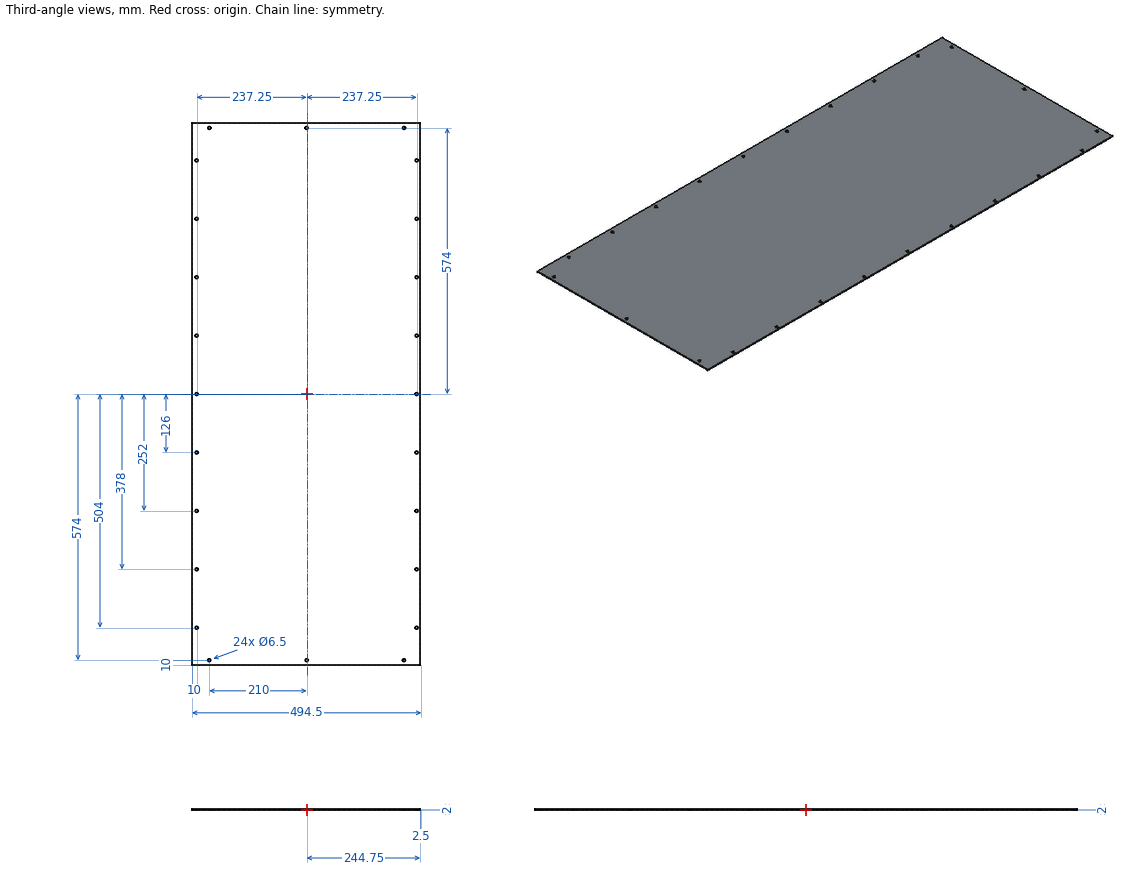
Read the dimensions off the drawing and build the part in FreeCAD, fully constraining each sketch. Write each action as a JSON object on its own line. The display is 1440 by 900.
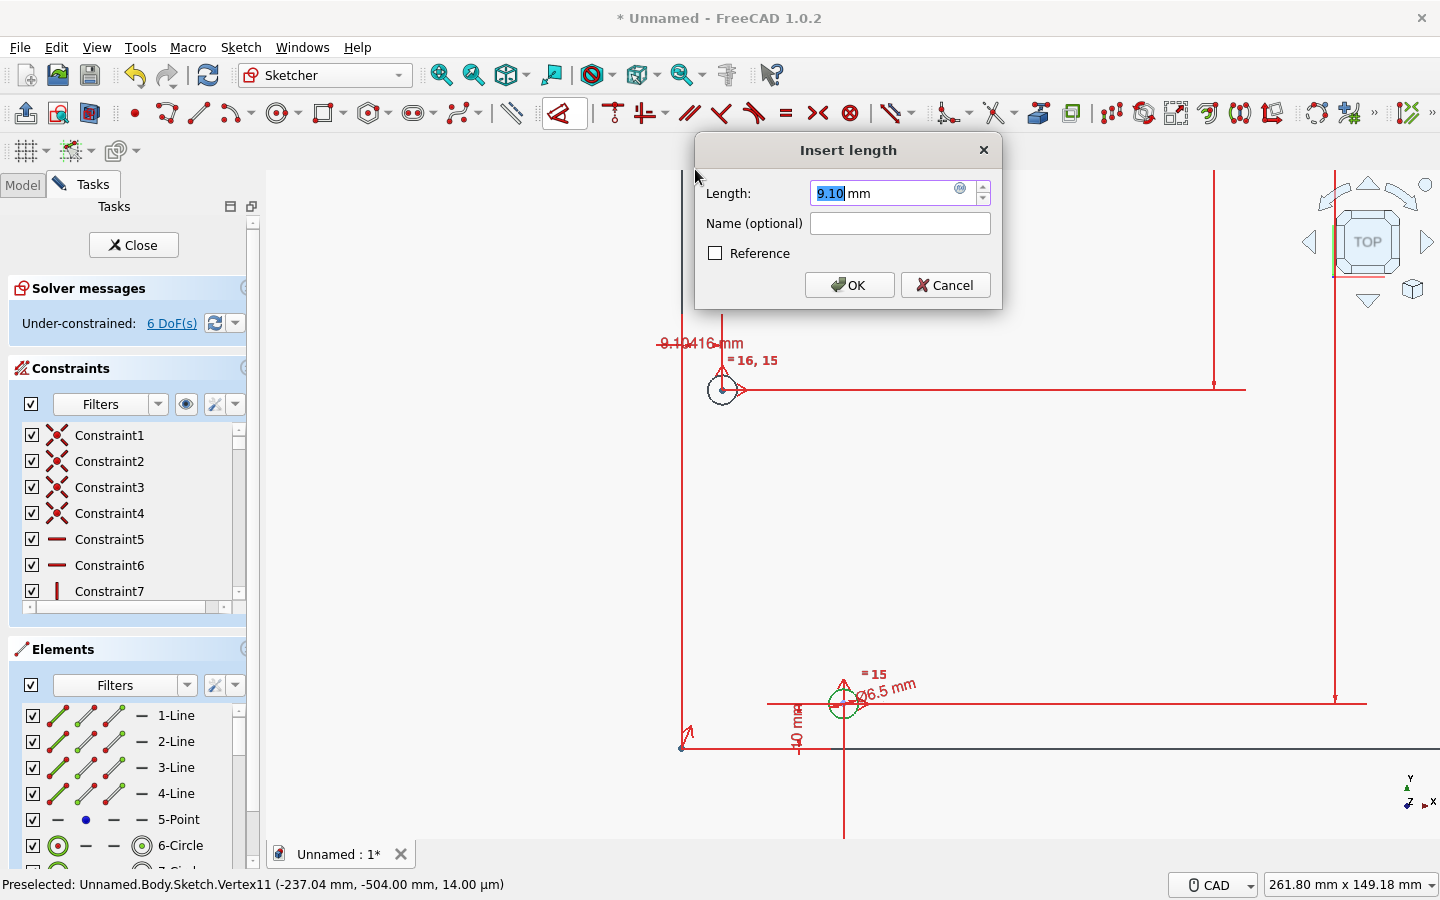
{"action": "type", "text": "10"}
{"action": "key", "text": "Return"}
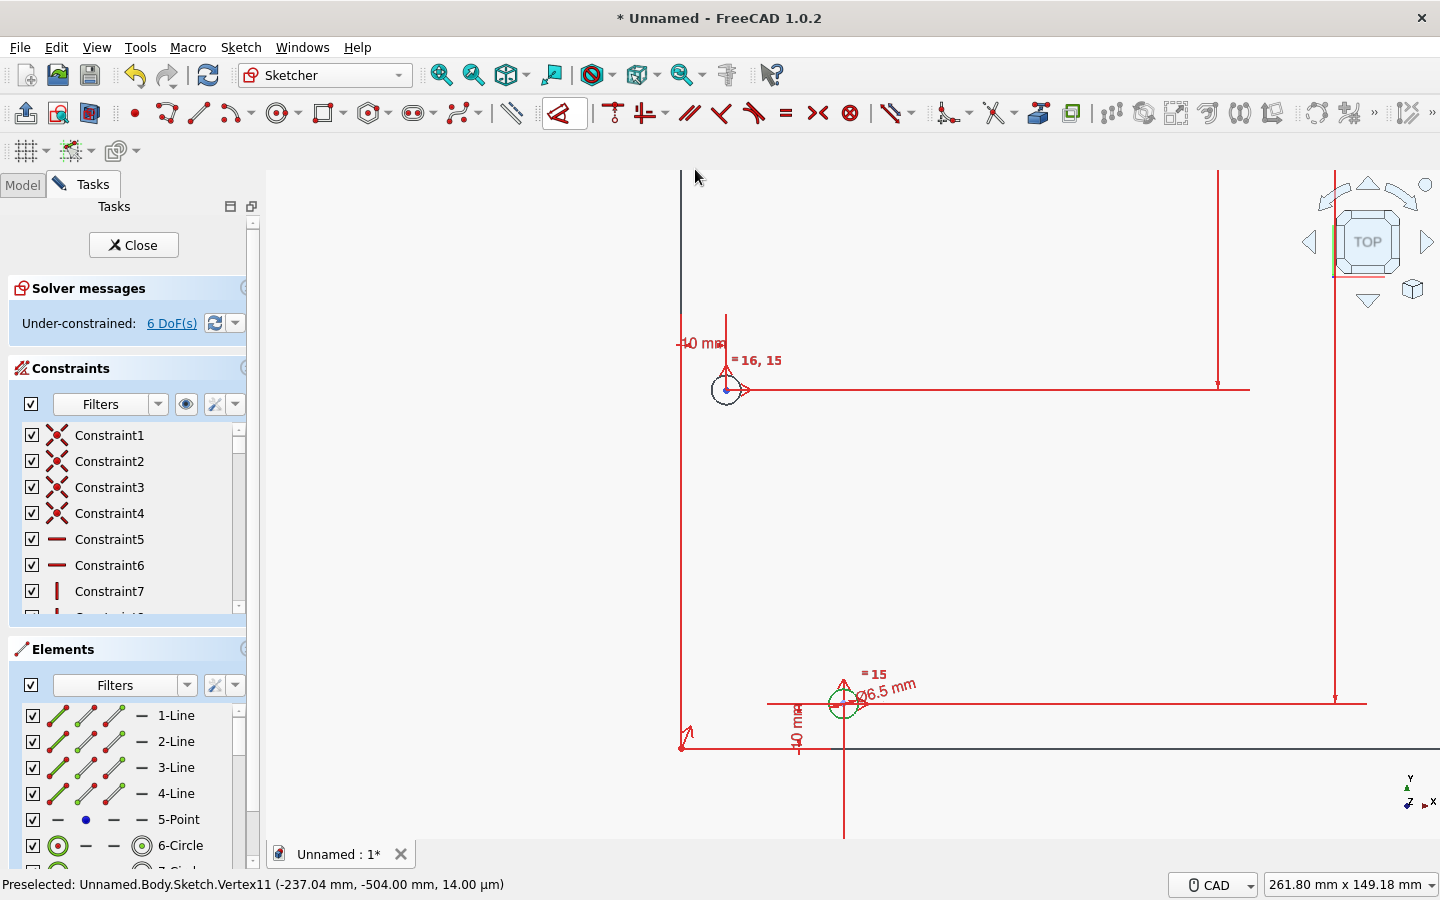
{"action": "left_click", "coordinate": [681, 749]}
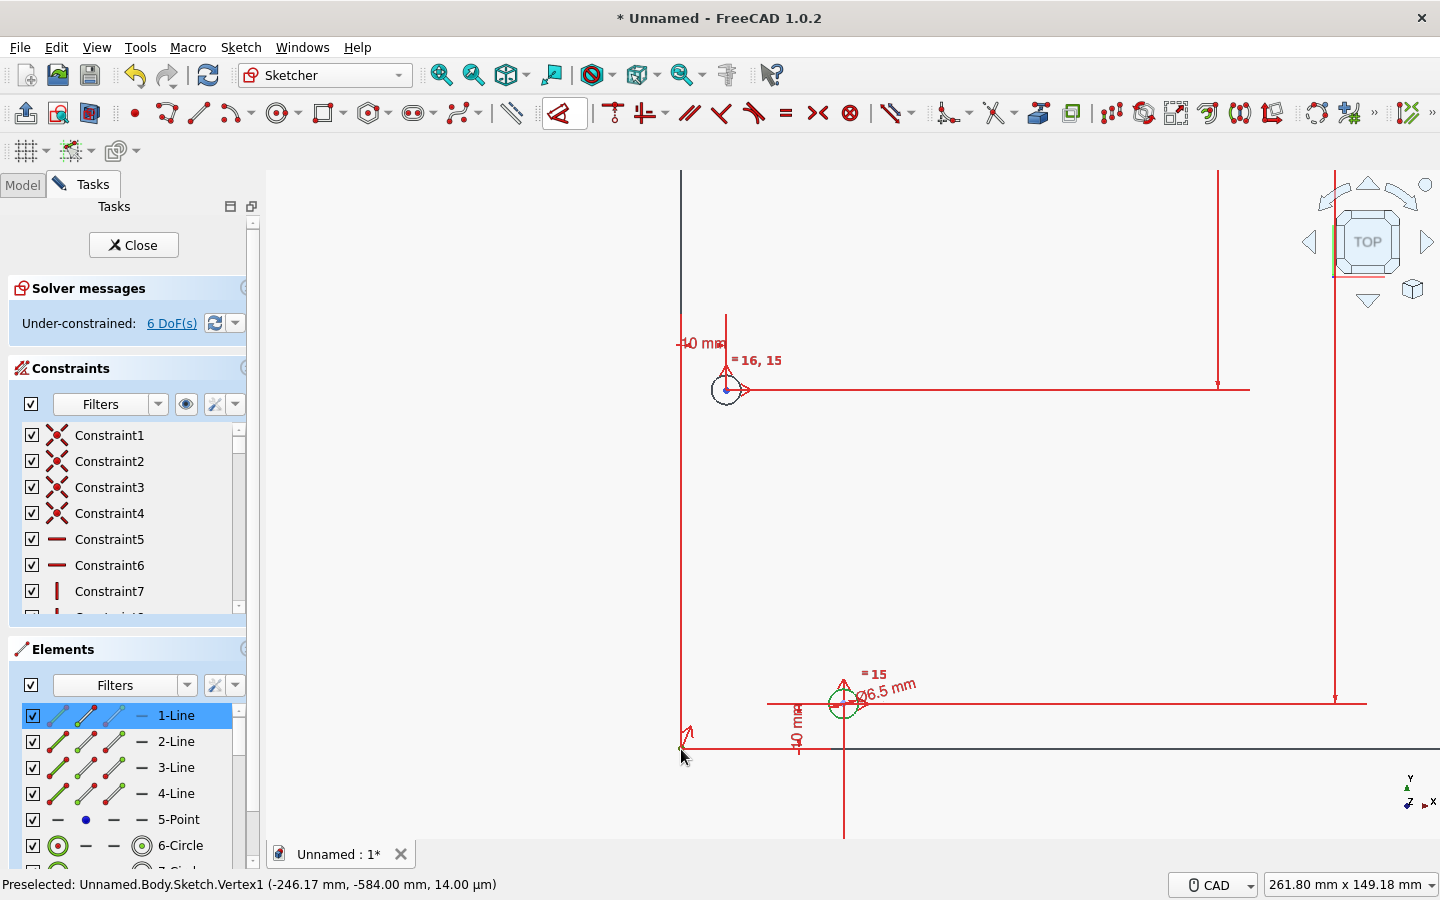
{"action": "scroll", "coordinate": [685, 741], "scroll_direction": "down", "scroll_amount": 12}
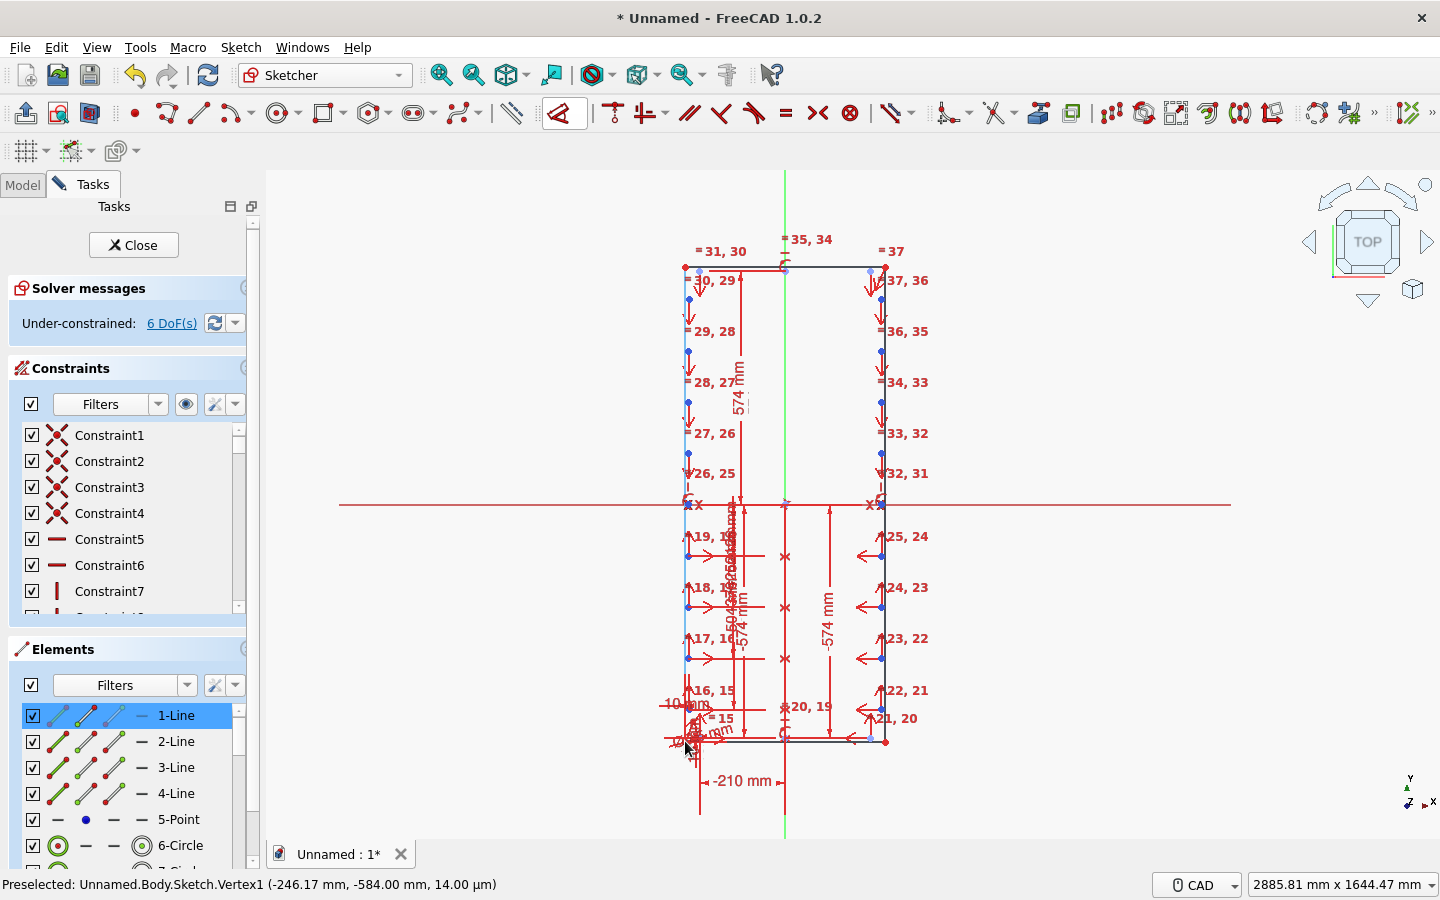
{"action": "scroll", "coordinate": [689, 659], "scroll_direction": "up", "scroll_amount": 12}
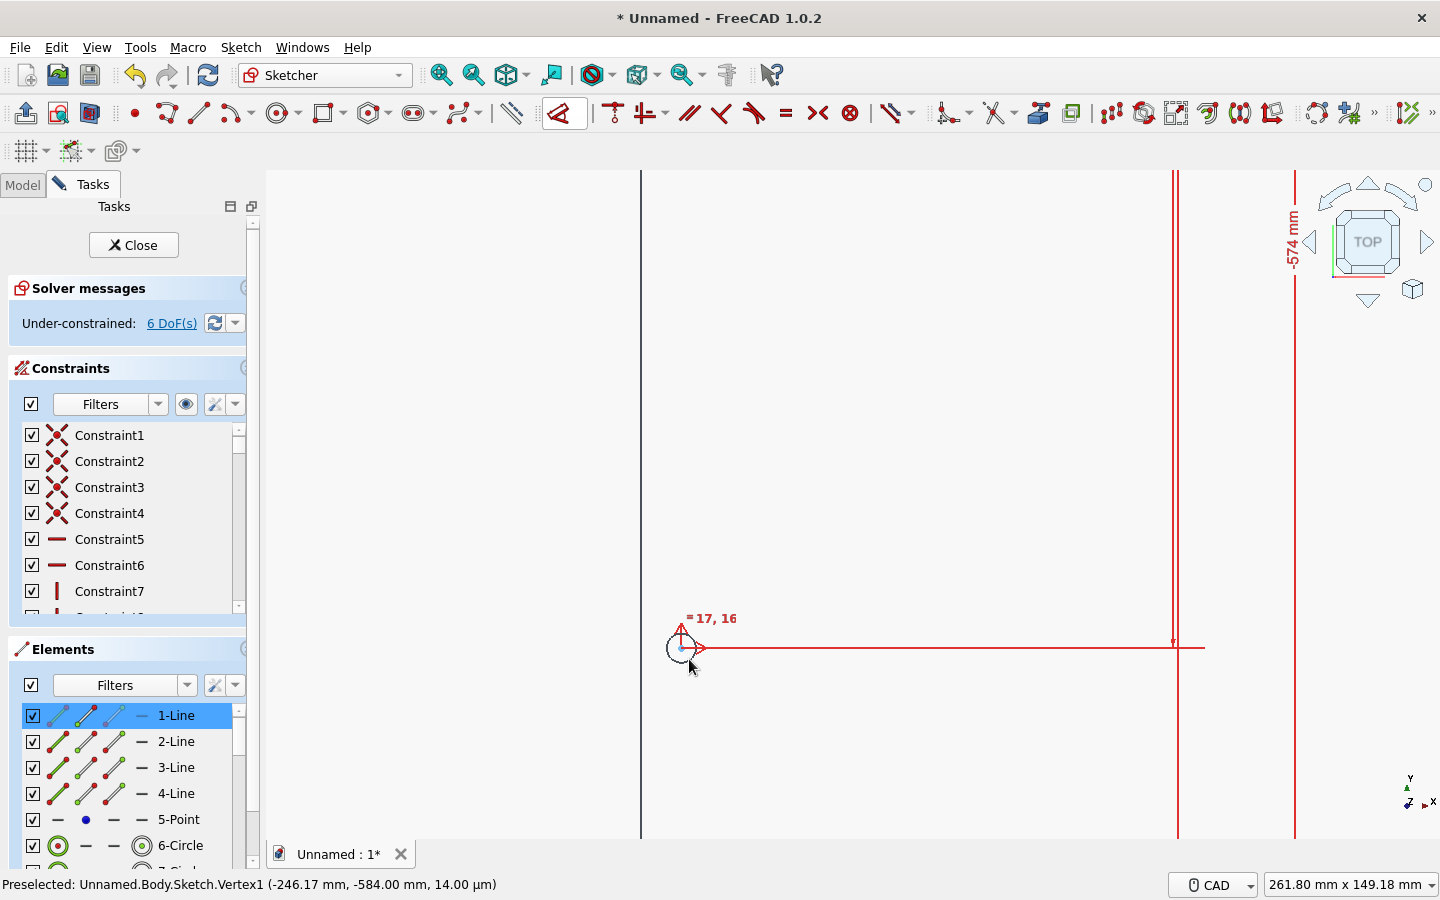
{"action": "left_click", "coordinate": [681, 648]}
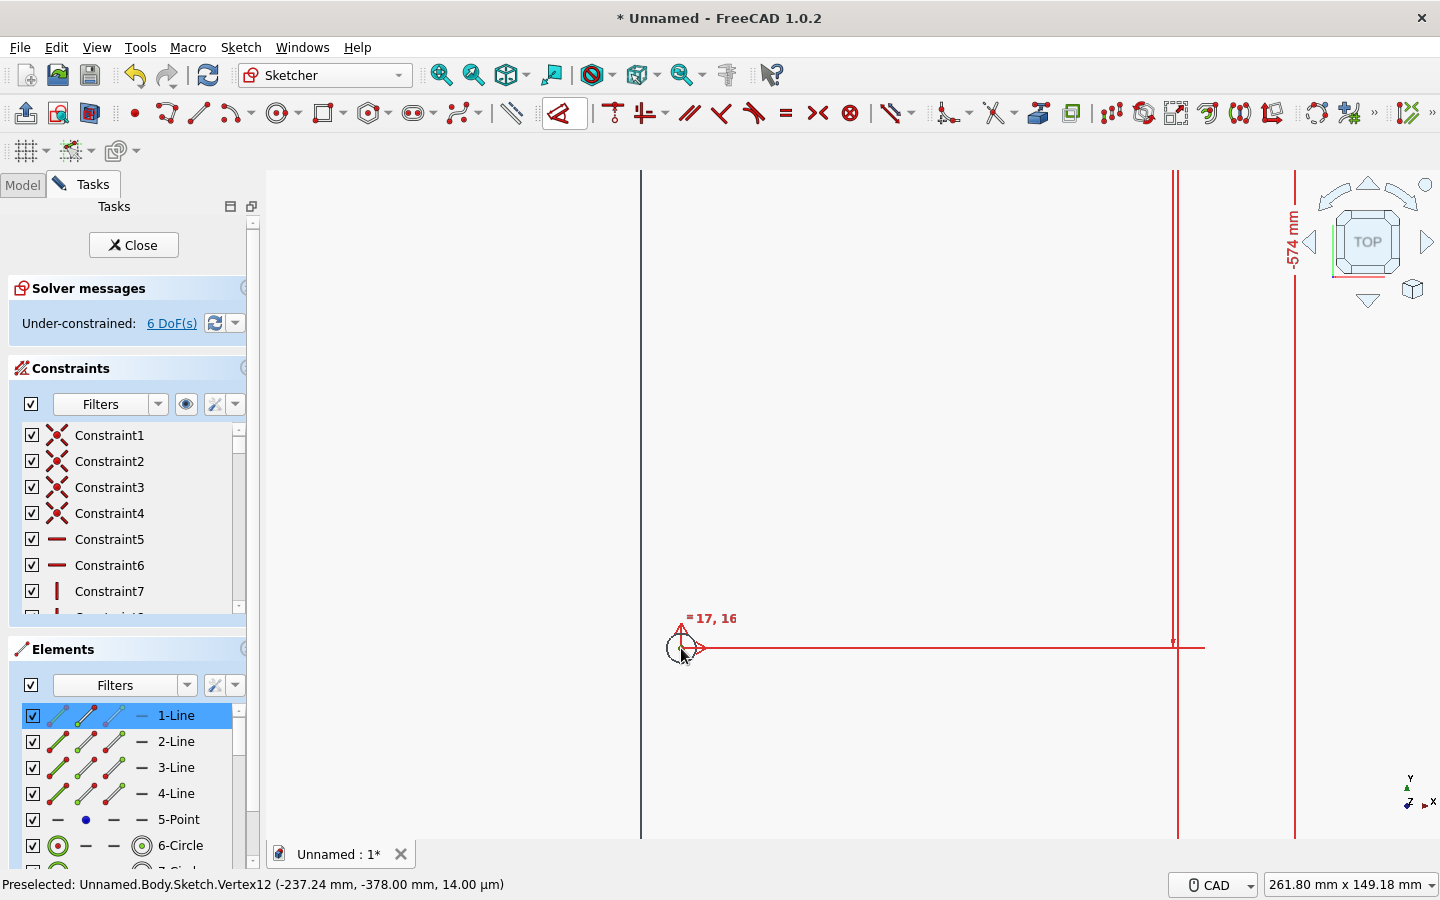
{"action": "key", "text": "l"}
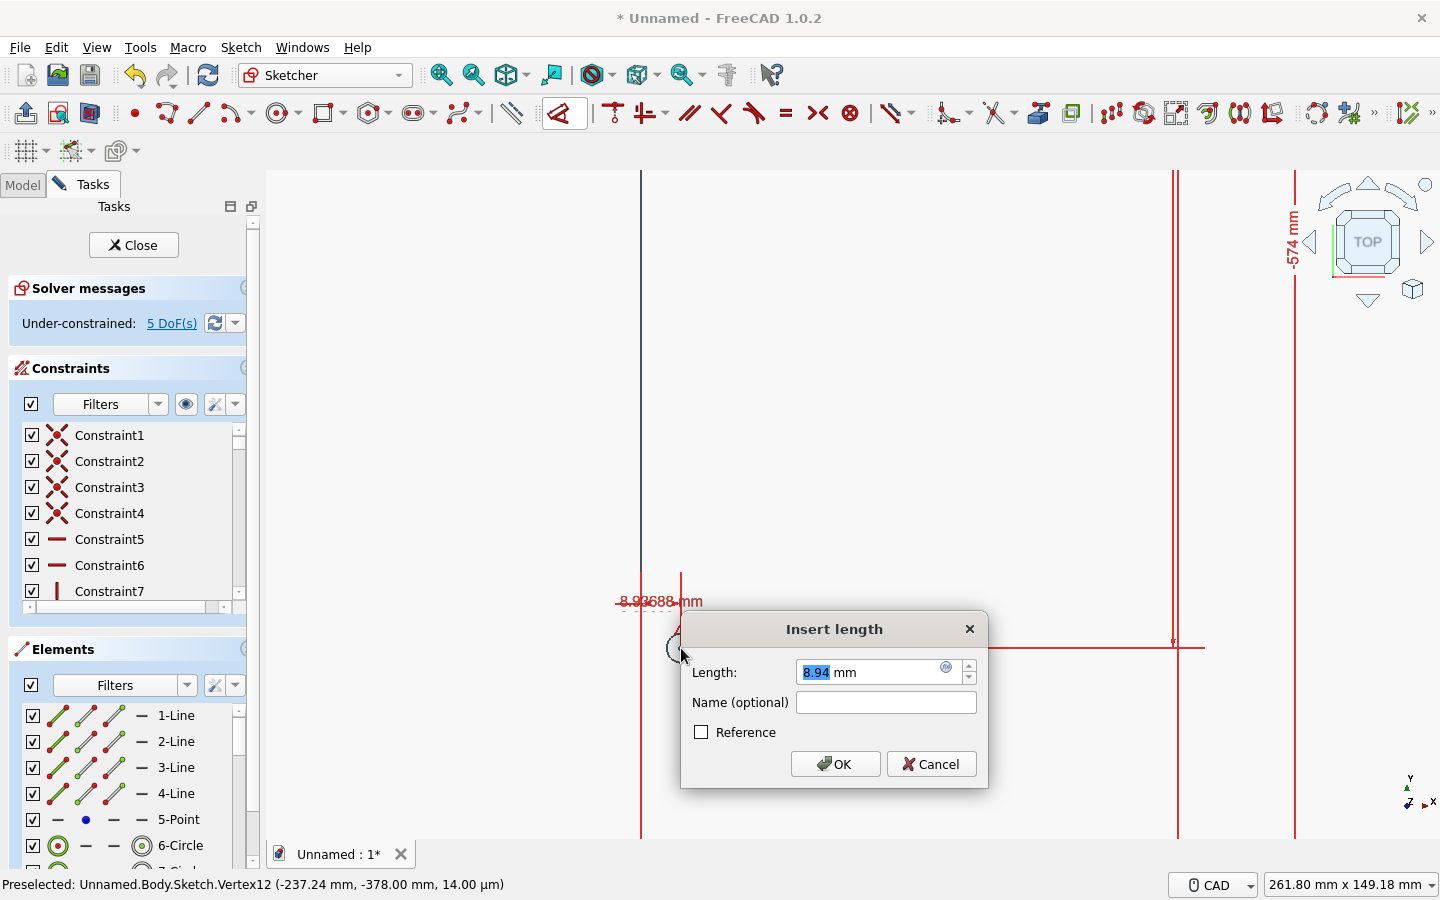
{"action": "type", "text": "10"}
{"action": "key", "text": "Return"}